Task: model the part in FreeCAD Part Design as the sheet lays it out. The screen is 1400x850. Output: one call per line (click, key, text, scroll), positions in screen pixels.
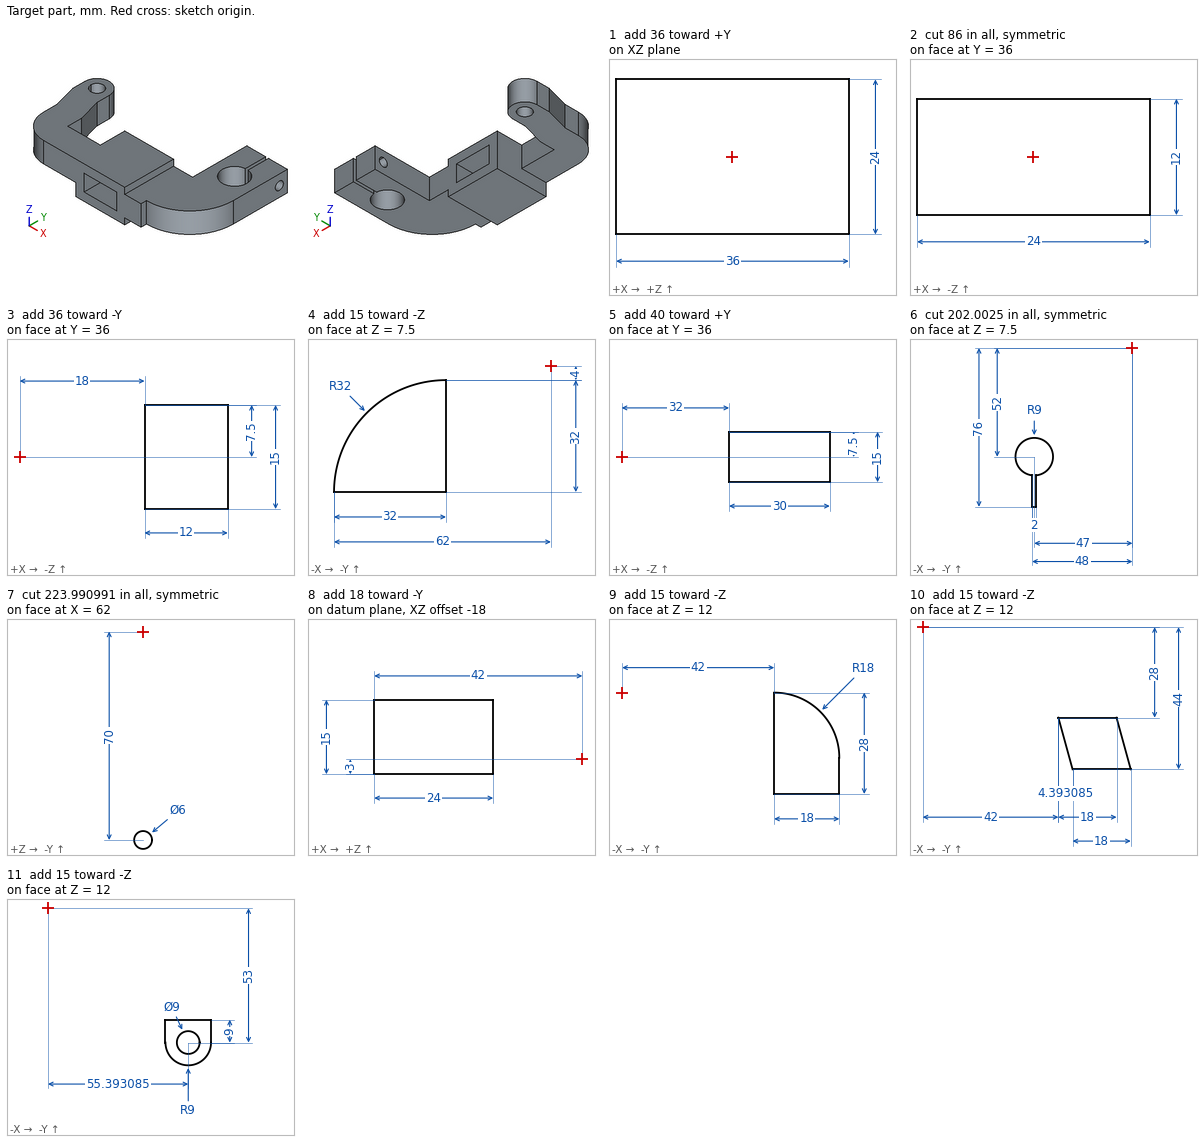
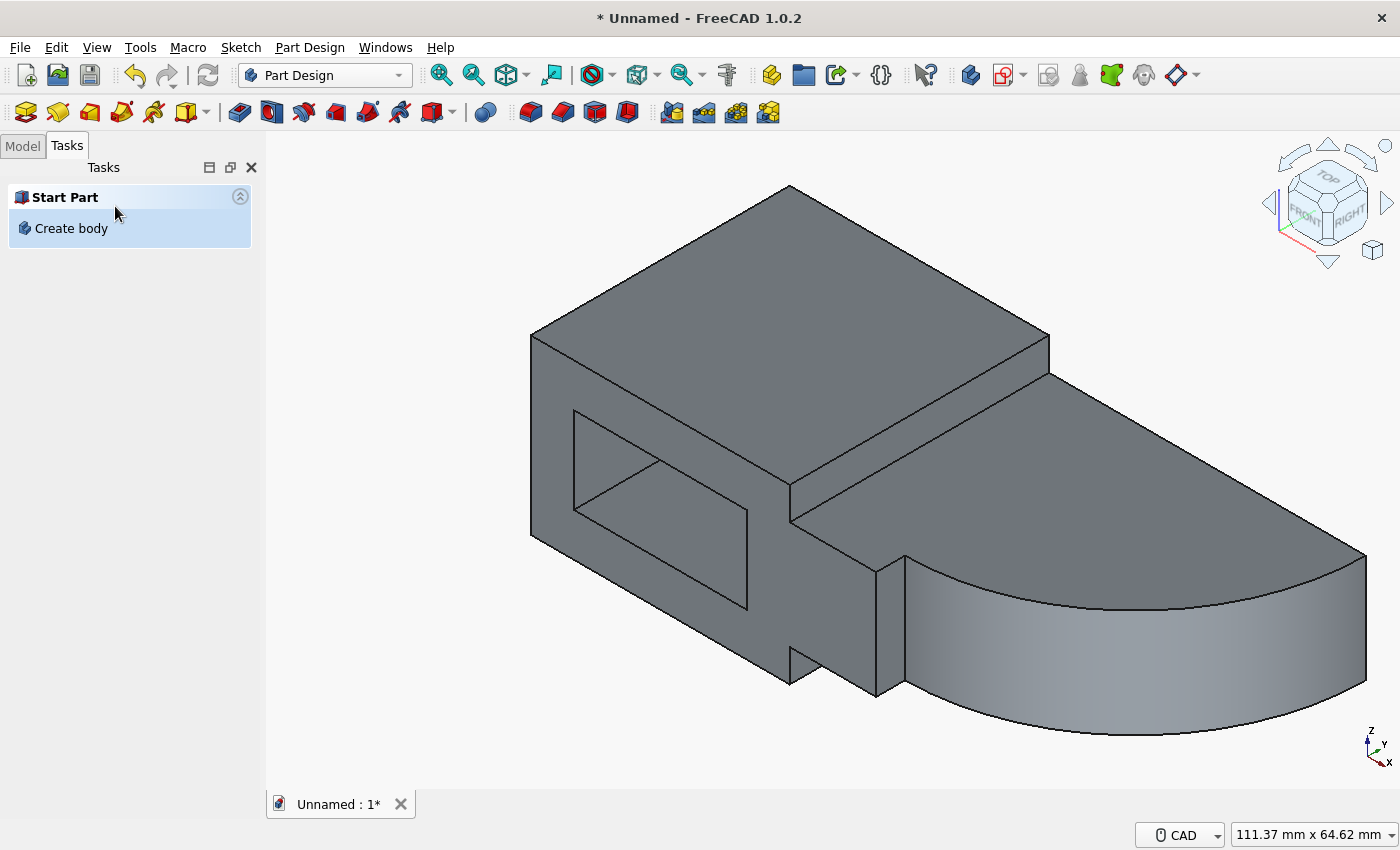
key(v)
key(f)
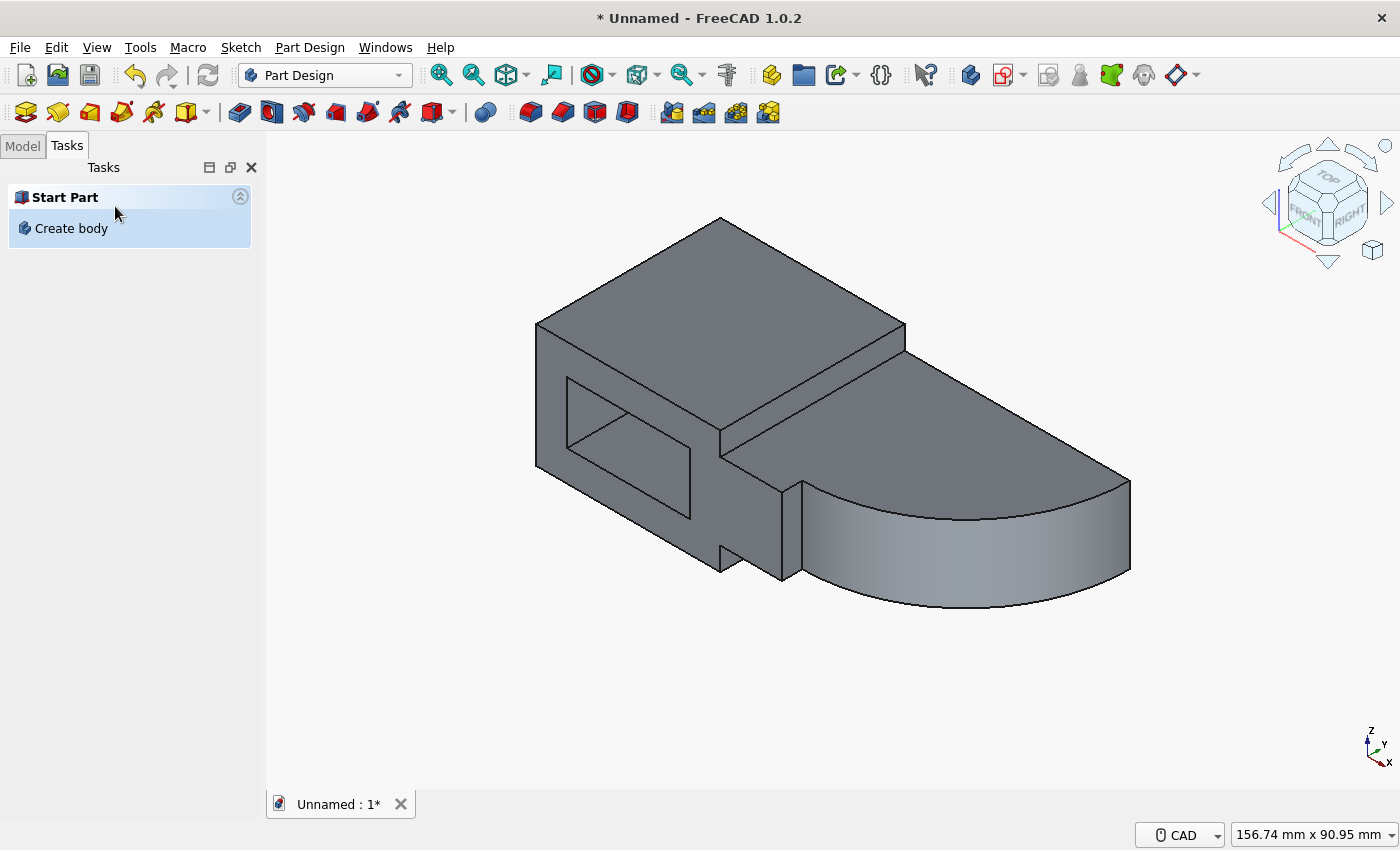
key(4)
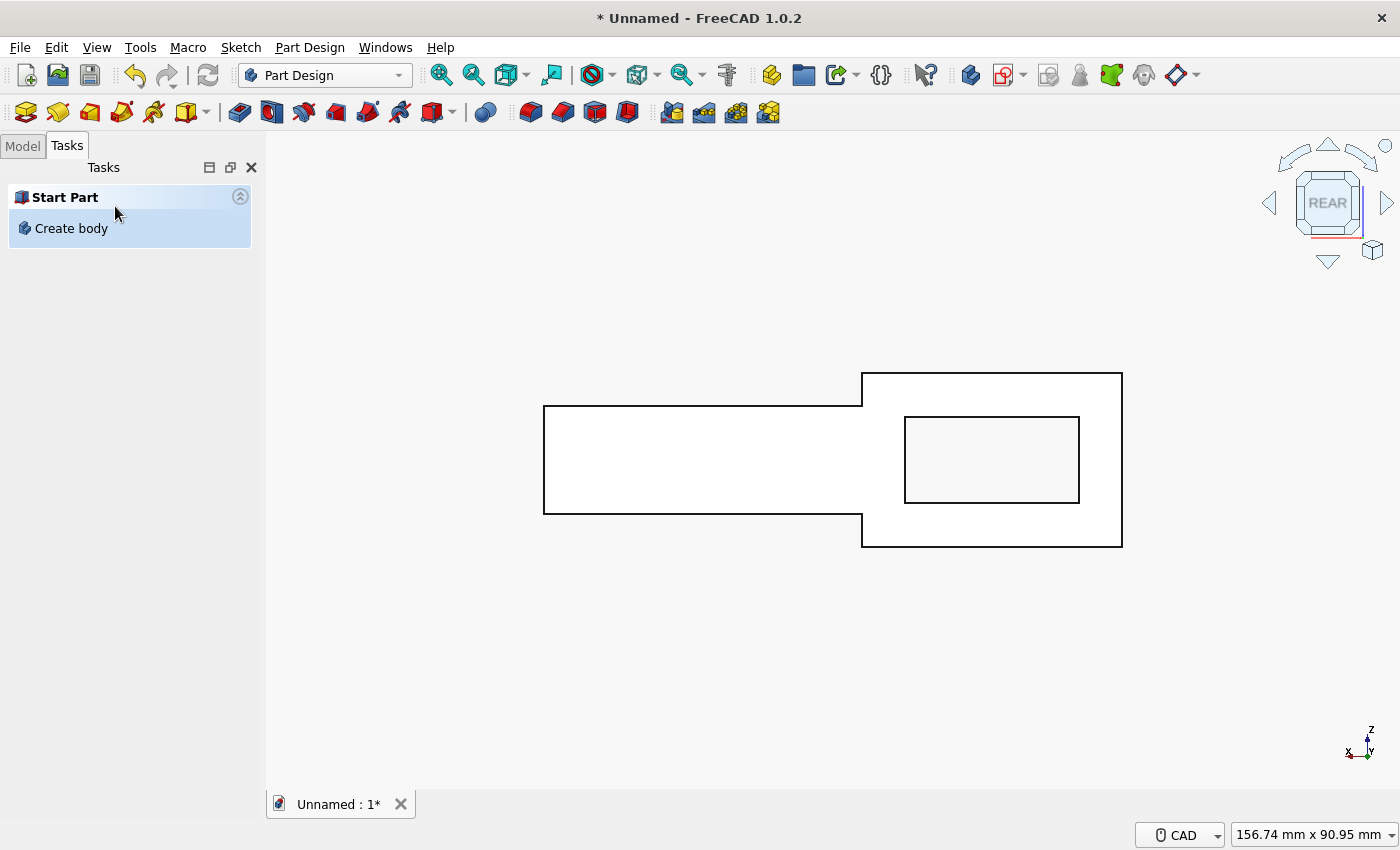
click(668, 459)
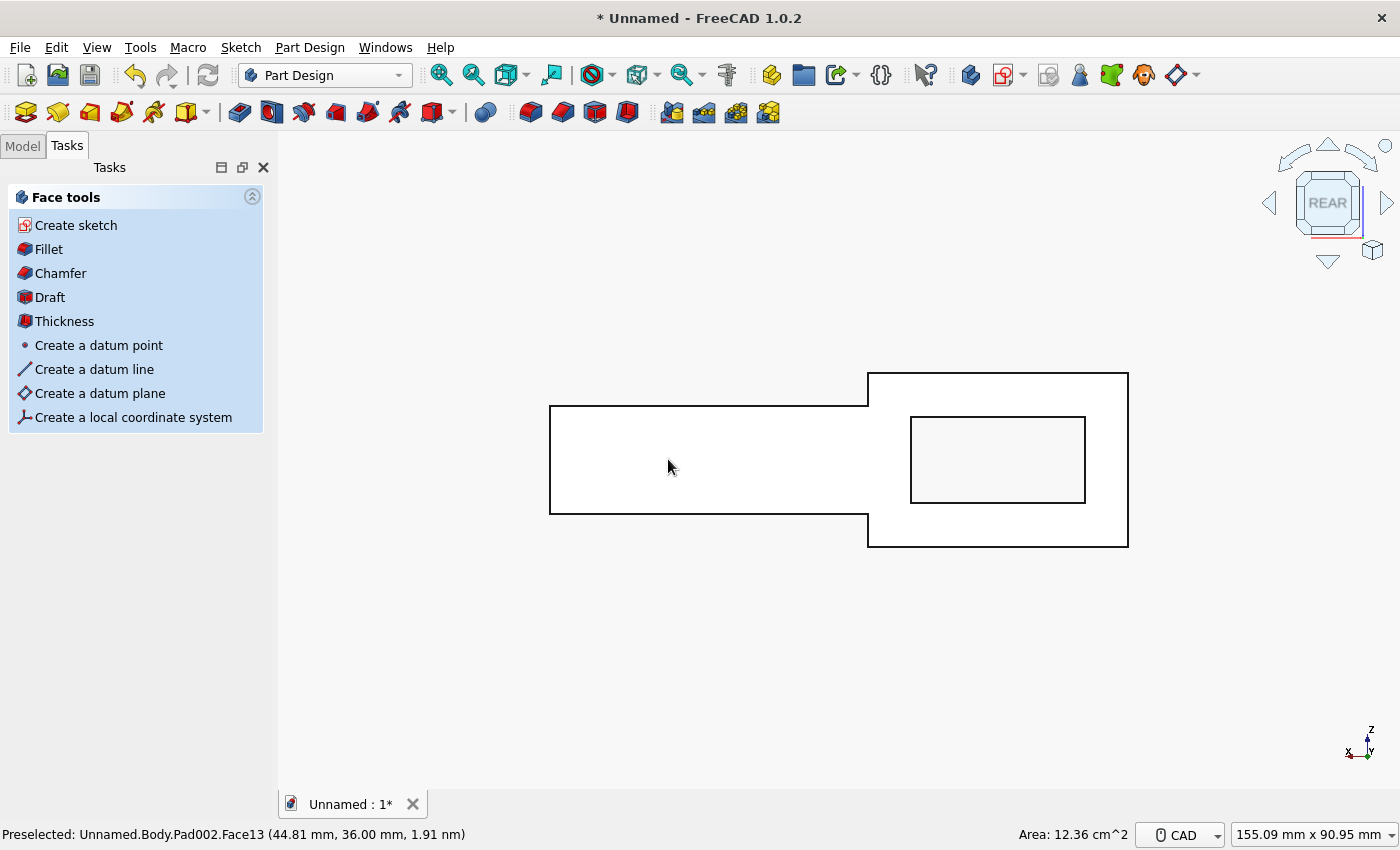
click(1004, 76)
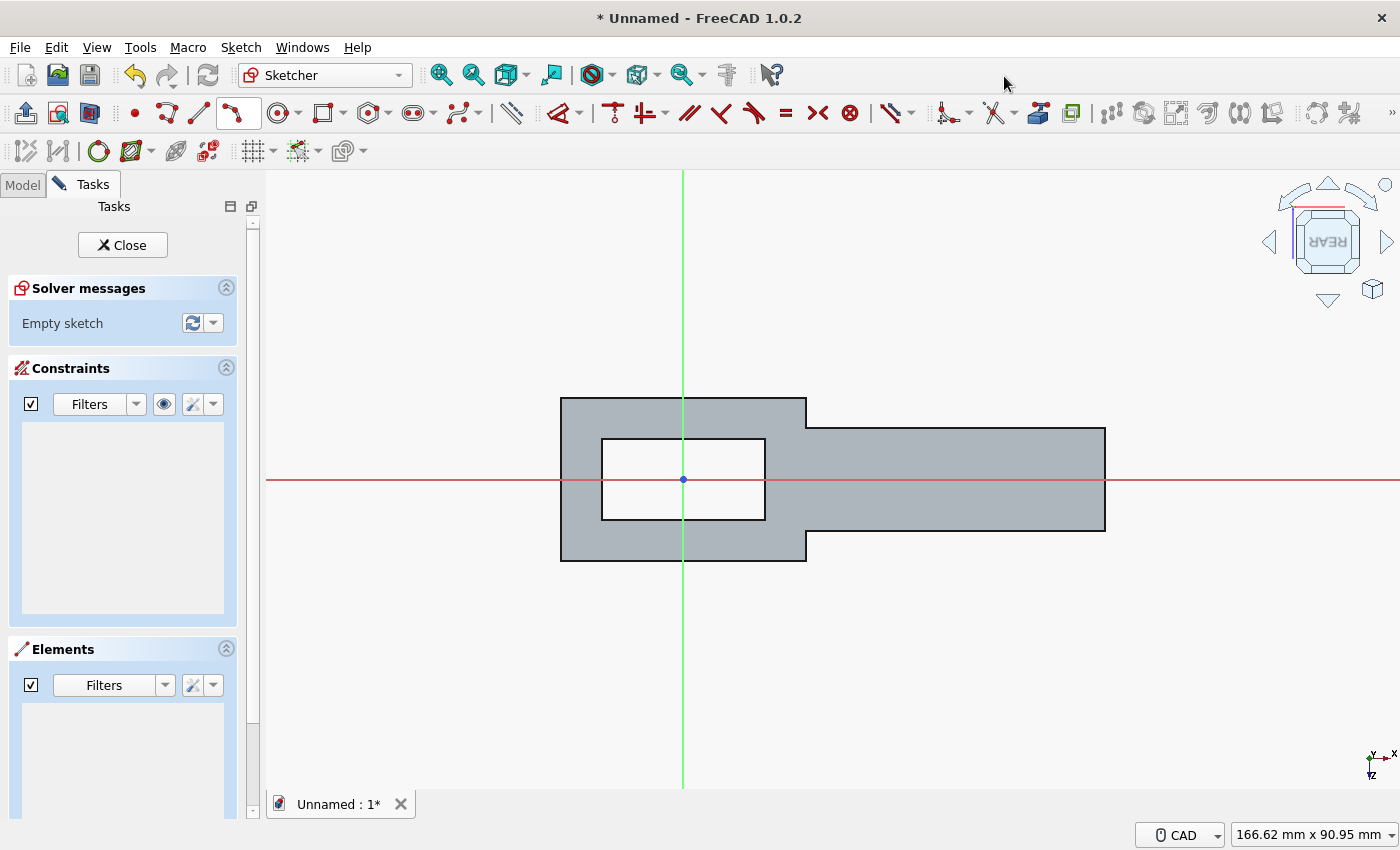
scroll(1158, 480, up, 2)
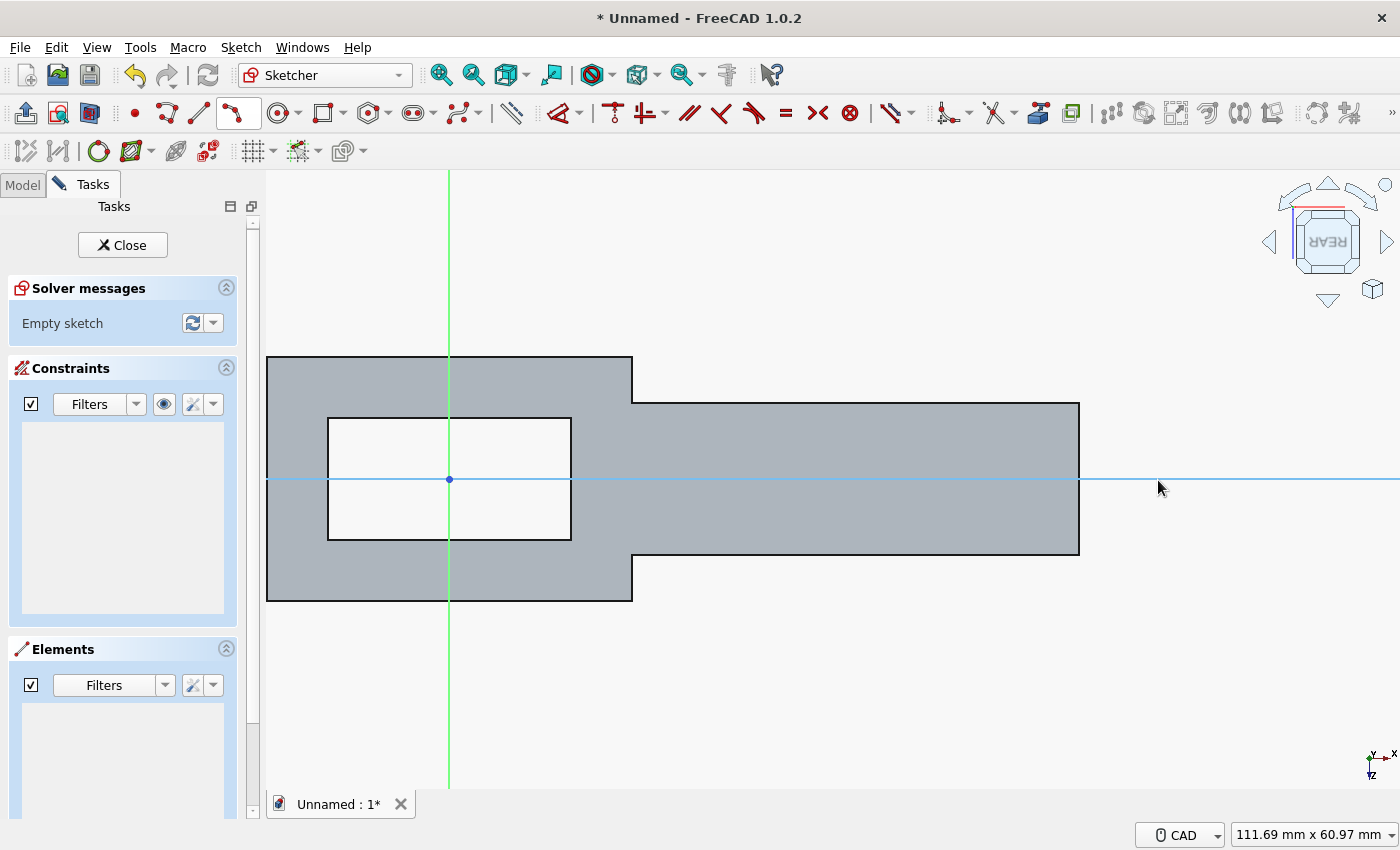
click(324, 114)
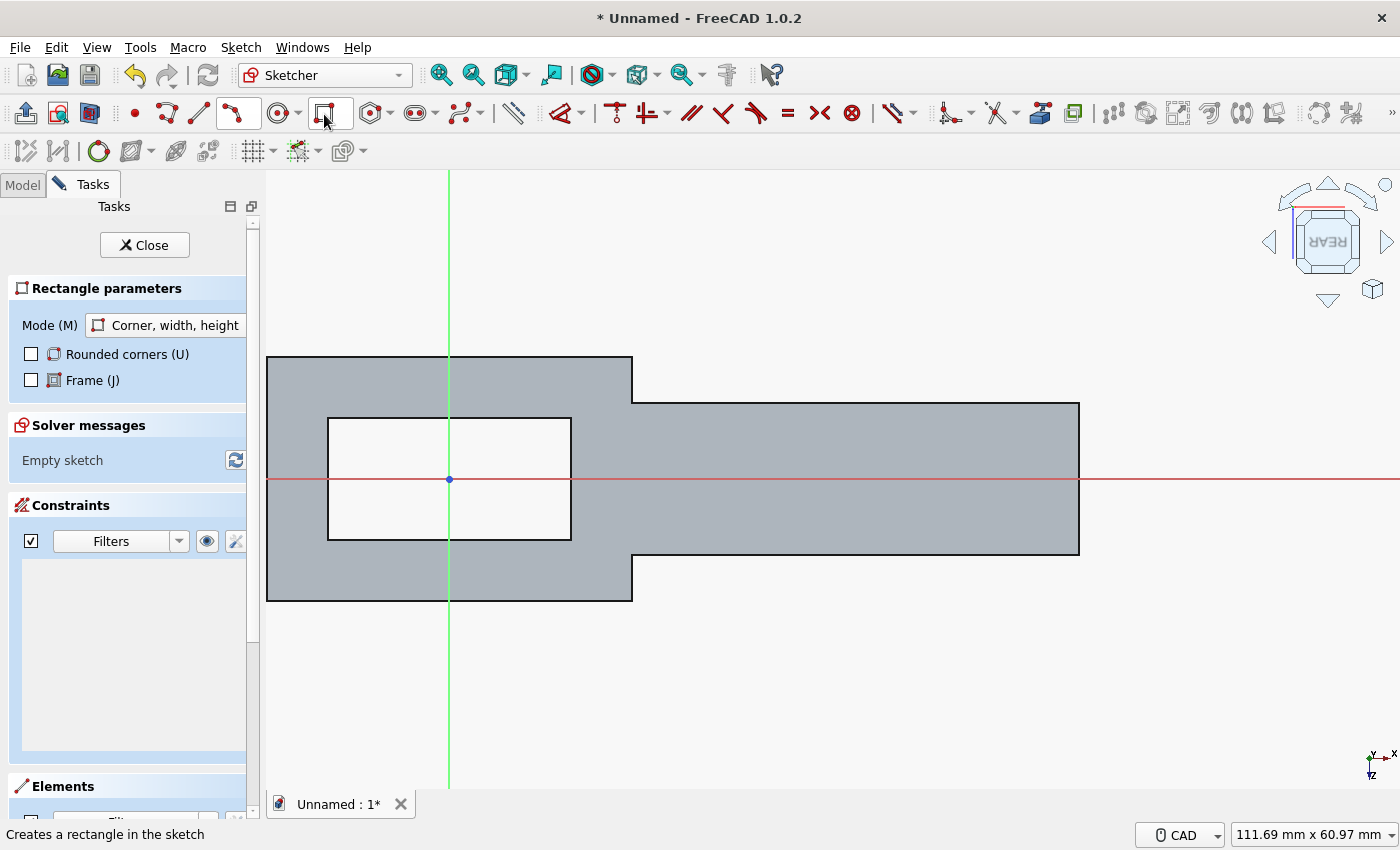
click(774, 403)
click(1079, 555)
key(Escape)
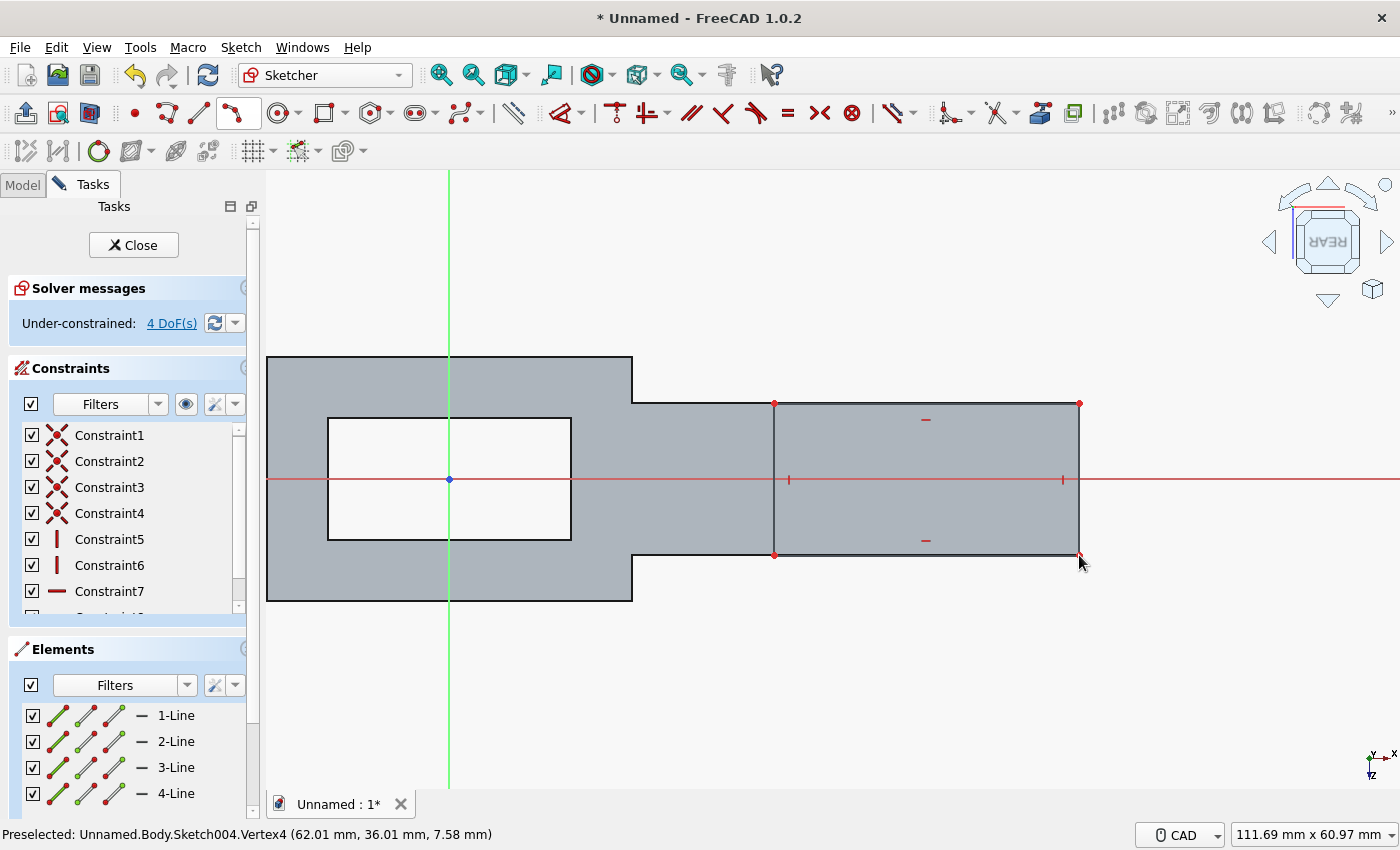
key(d)